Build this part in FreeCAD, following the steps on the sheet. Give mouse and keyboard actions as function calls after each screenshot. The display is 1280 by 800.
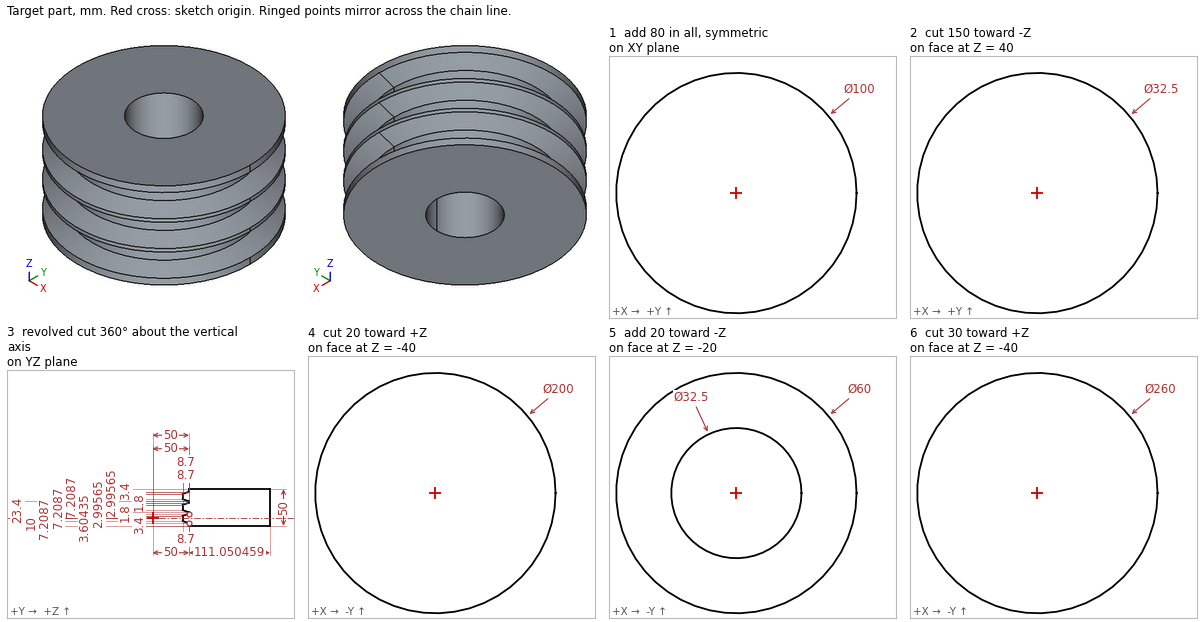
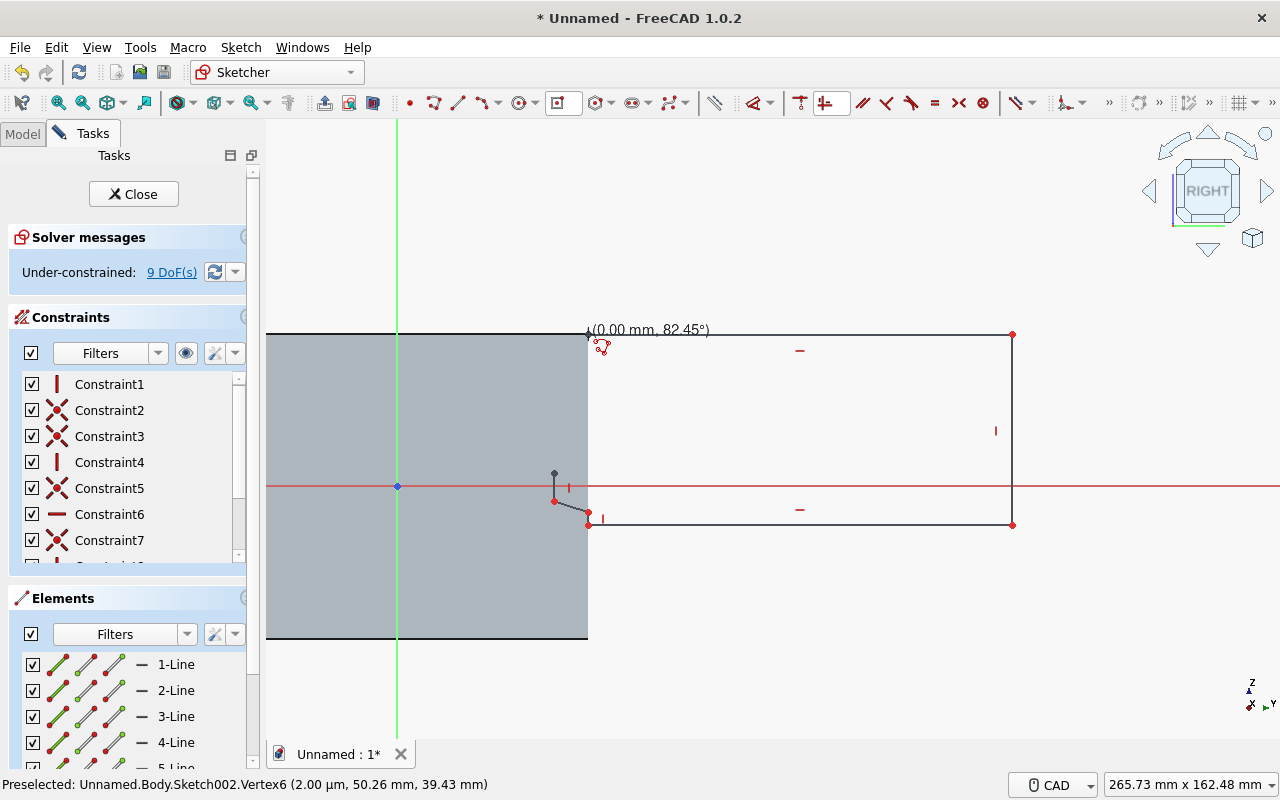
scroll(588, 347, up, 2)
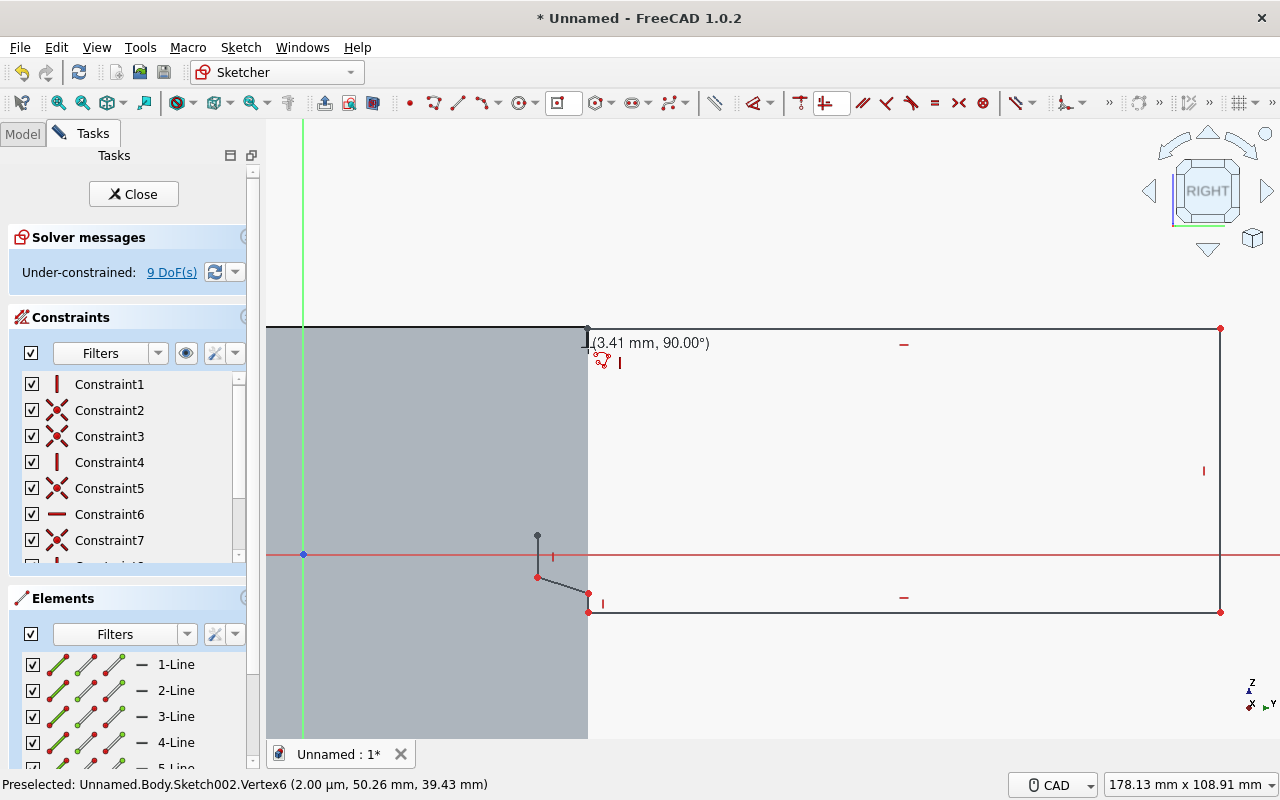
click(588, 347)
click(538, 364)
click(538, 405)
click(588, 422)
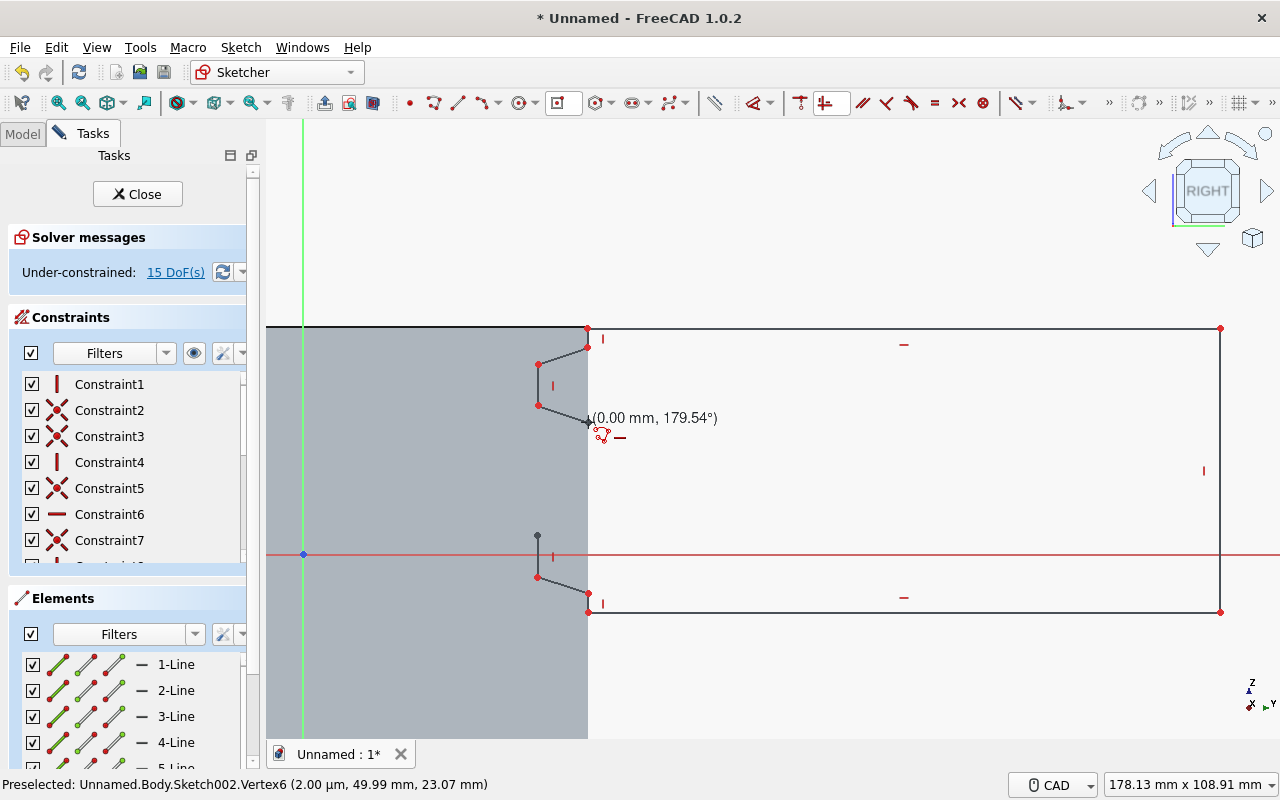
scroll(588, 432, up, 3)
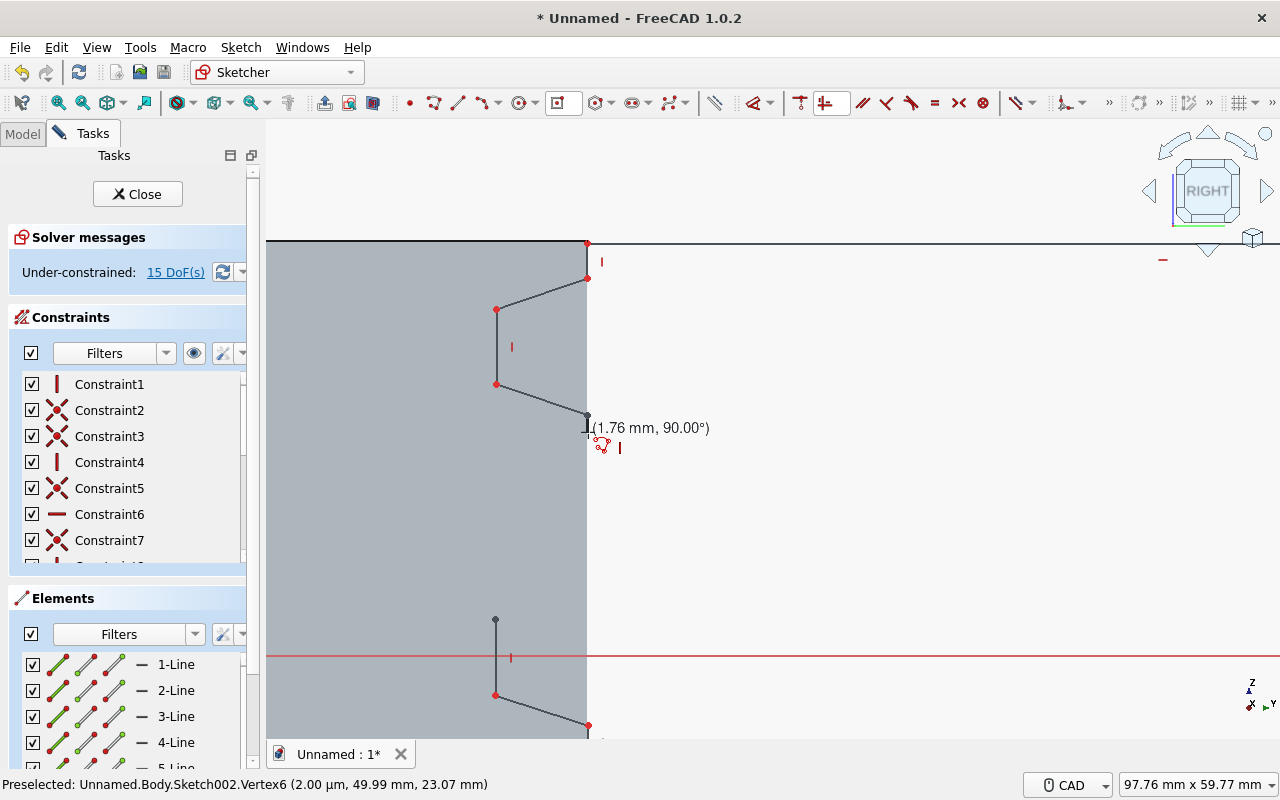
click(588, 431)
click(497, 463)
click(497, 537)
click(587, 568)
click(587, 587)
click(496, 620)
key(Escape)
key(Escape)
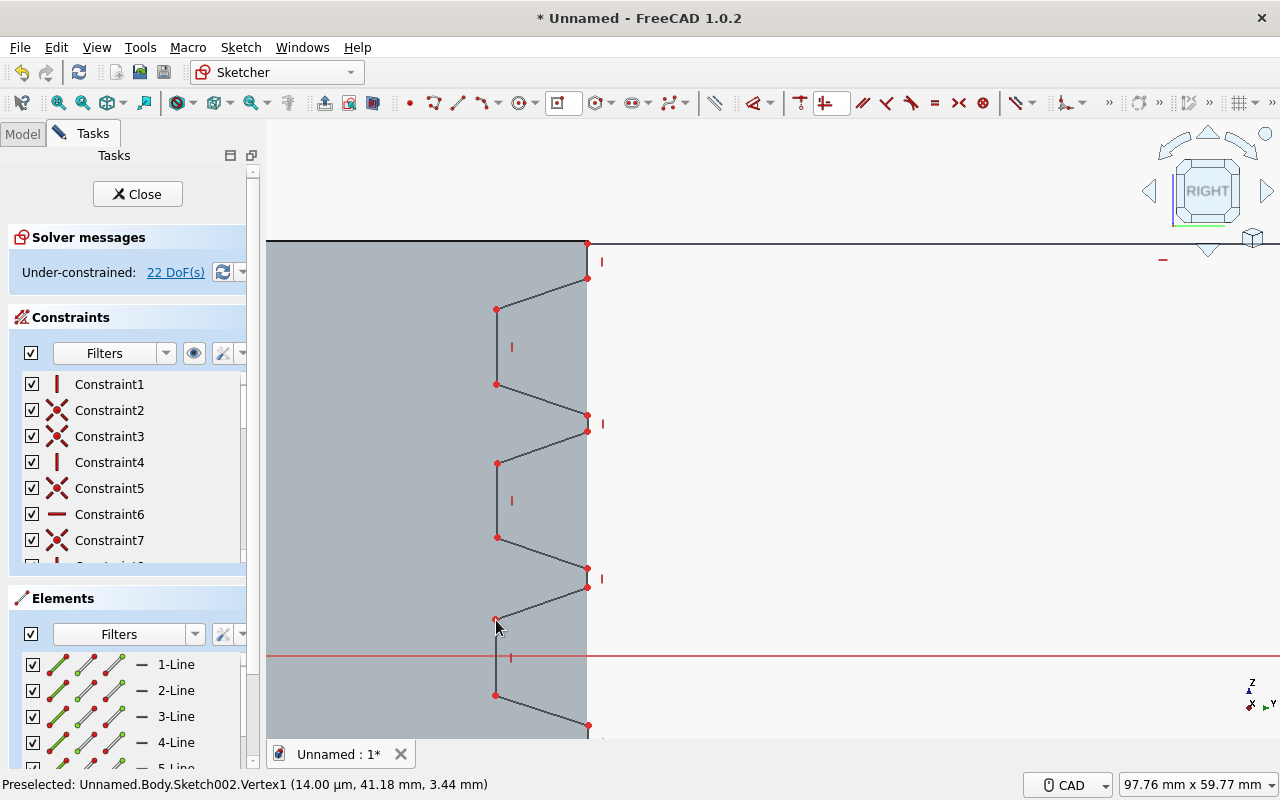
scroll(588, 388, down, 5)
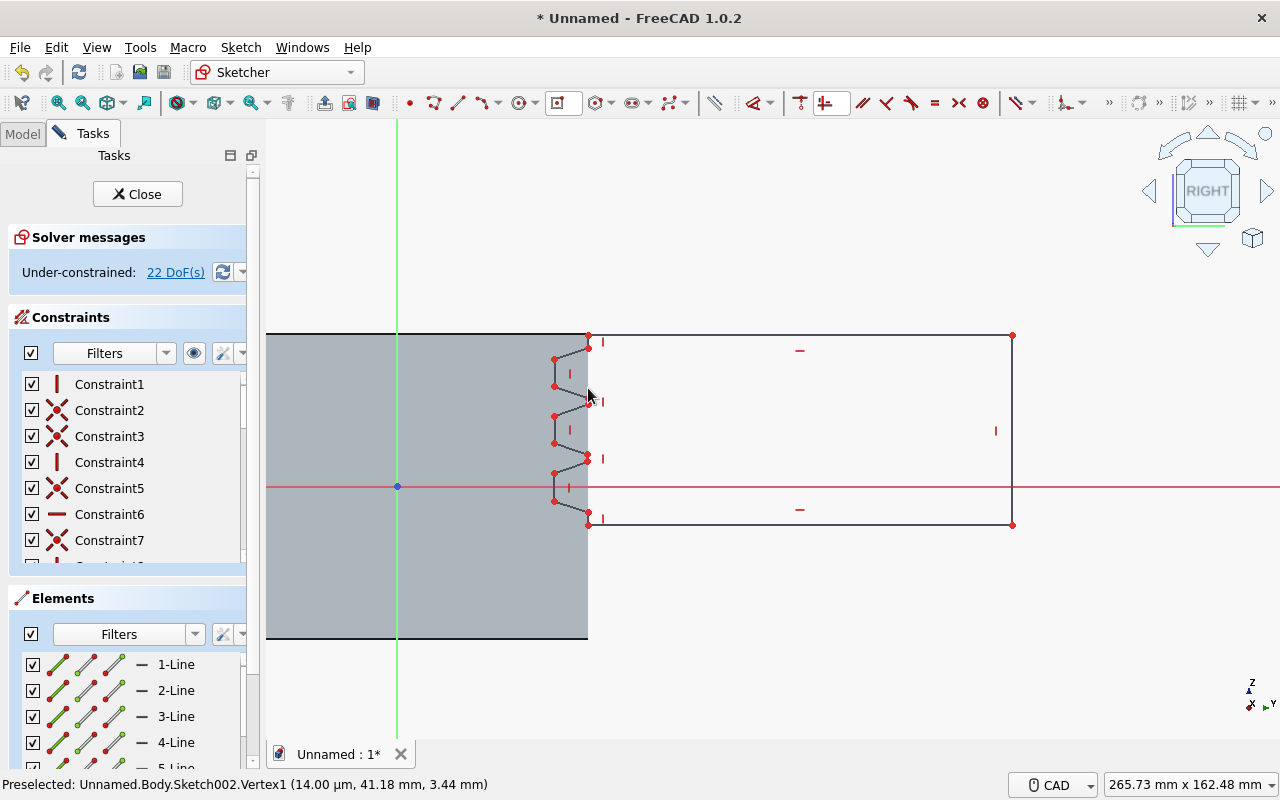
click(588, 513)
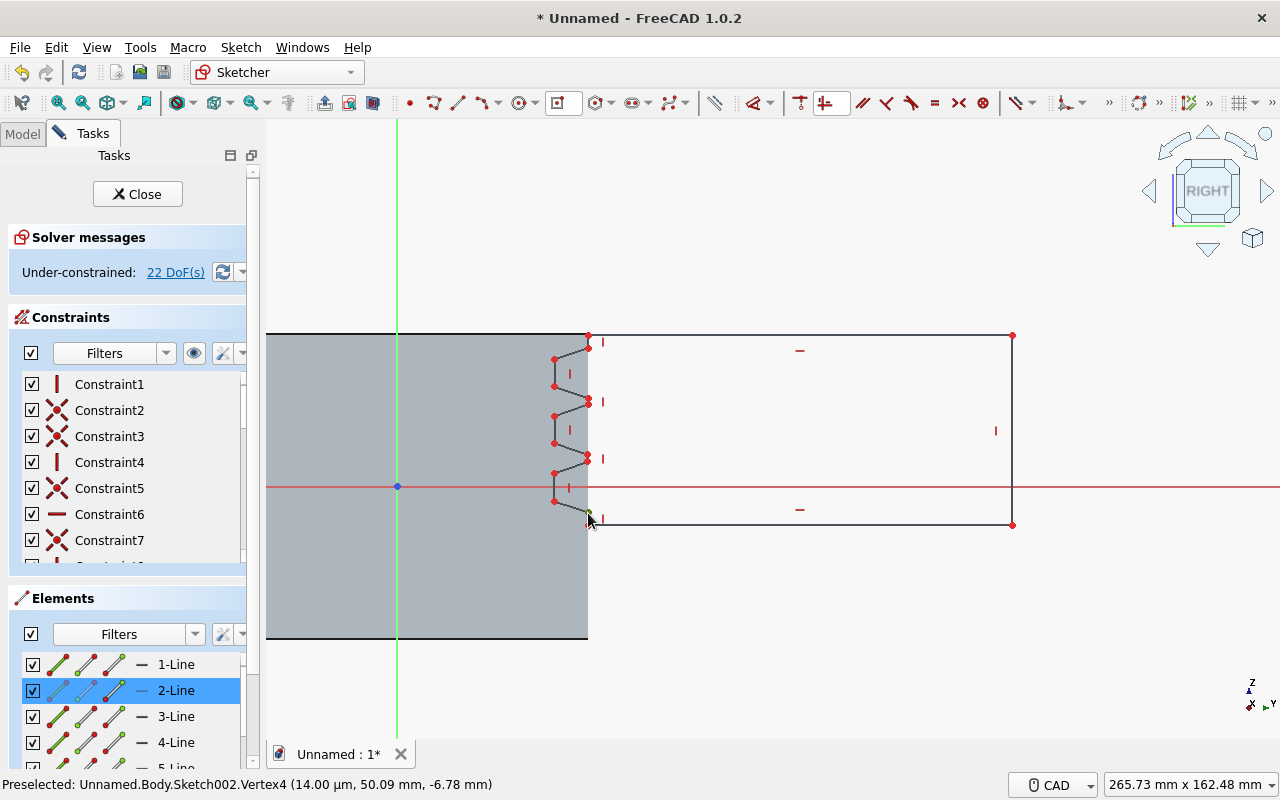
scroll(588, 462, up, 3)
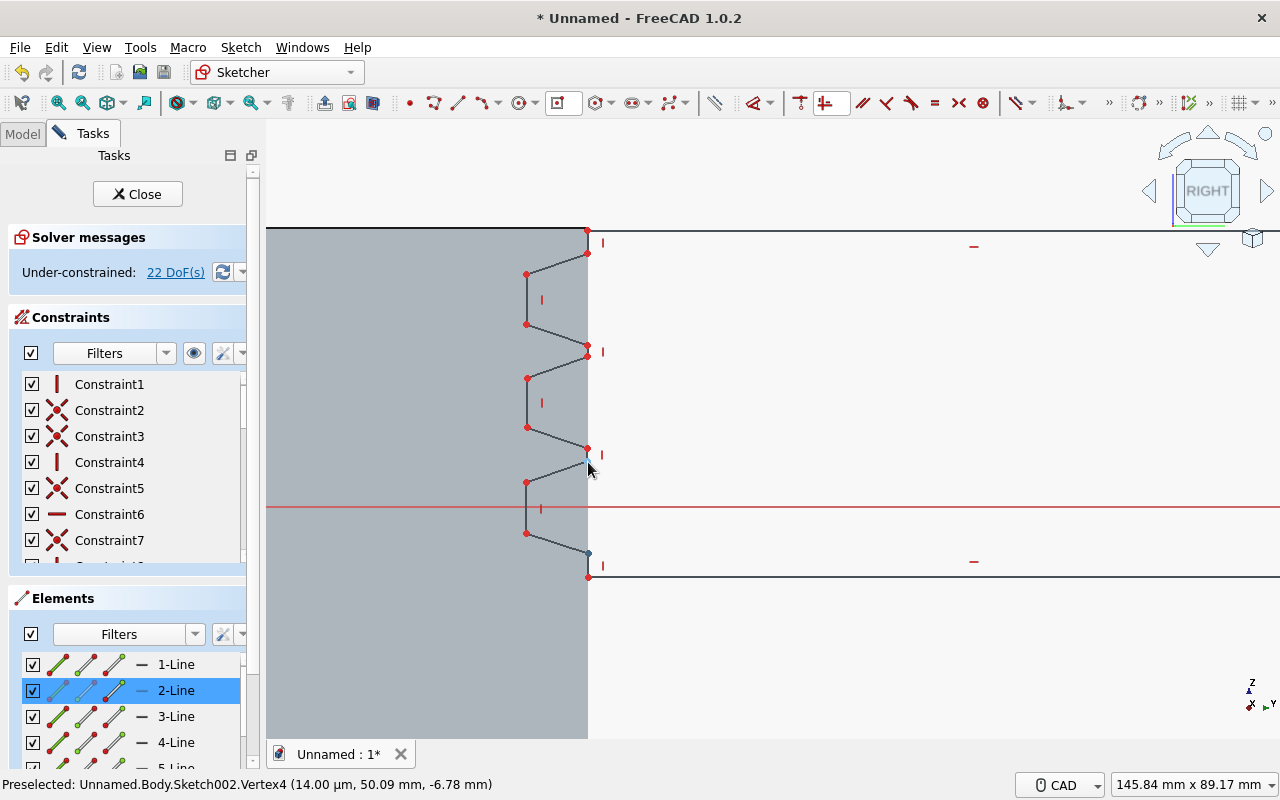
click(587, 461)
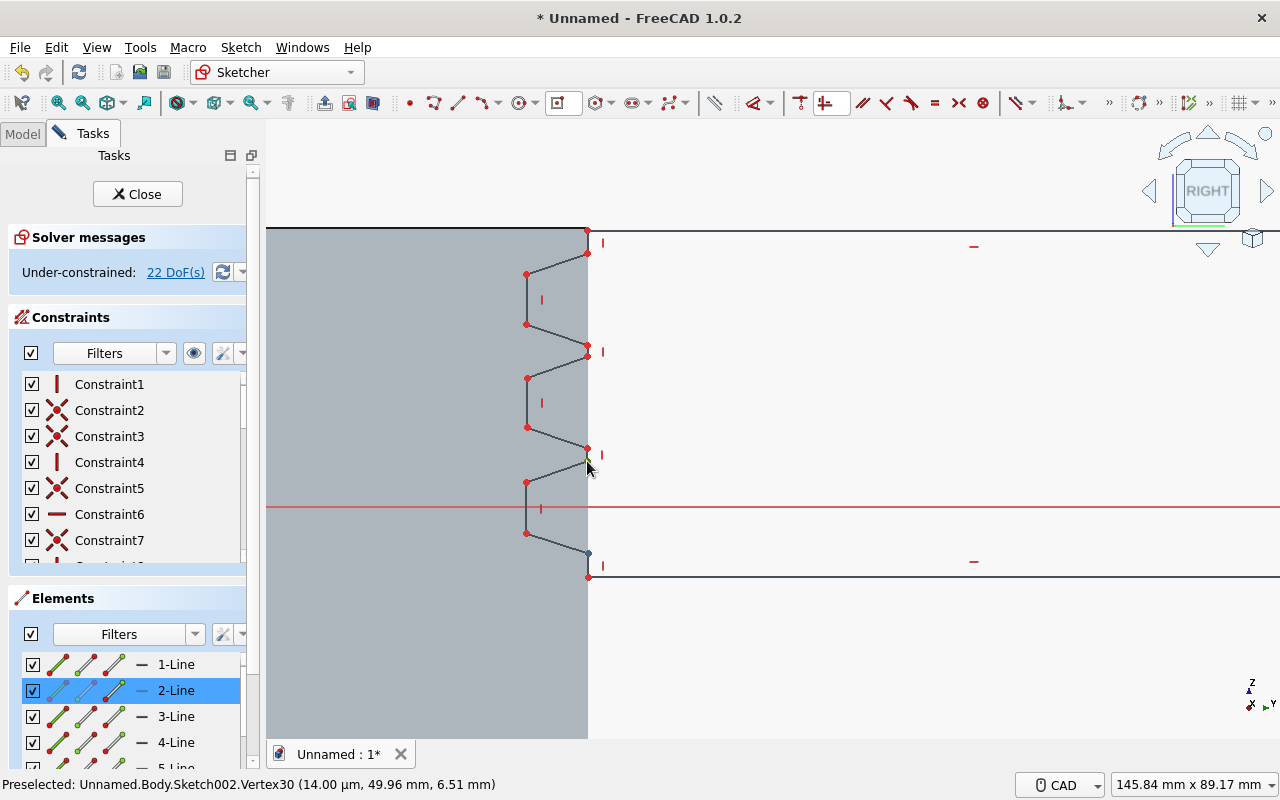
click(353, 507)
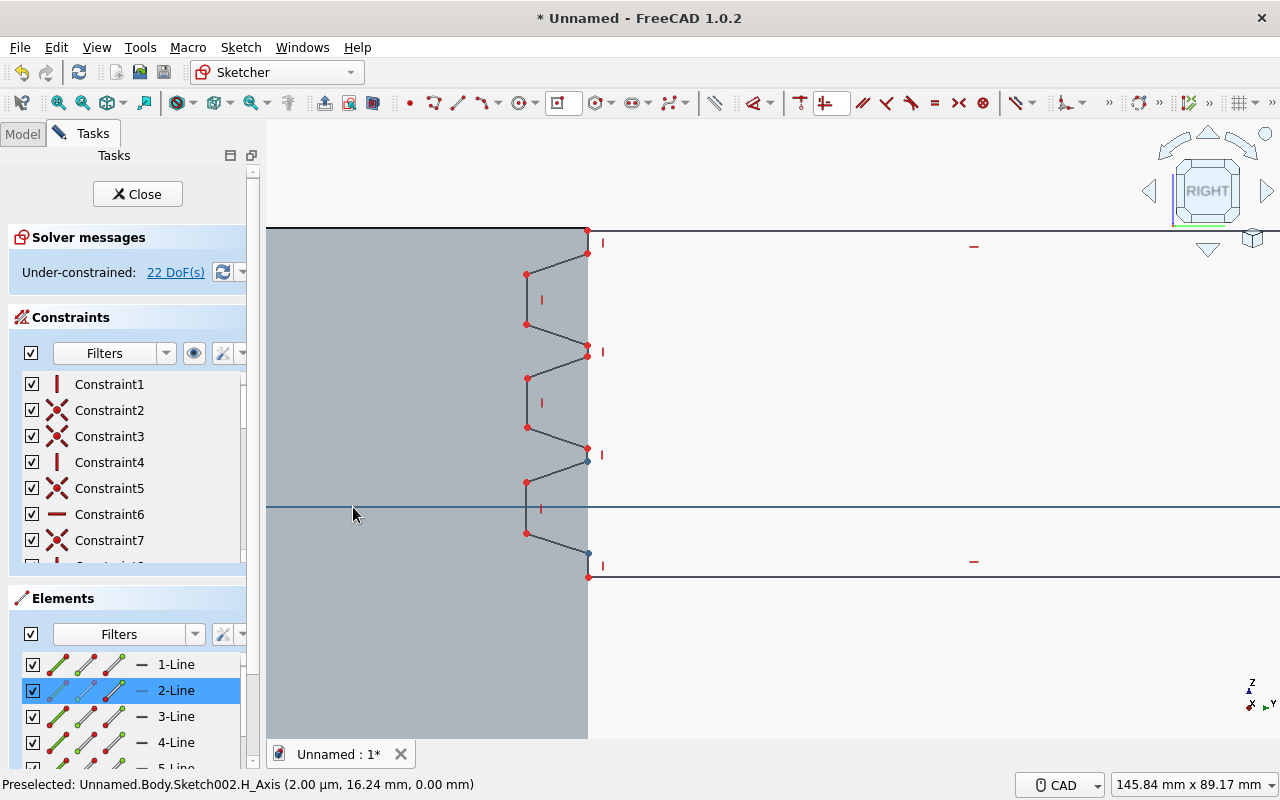
click(960, 104)